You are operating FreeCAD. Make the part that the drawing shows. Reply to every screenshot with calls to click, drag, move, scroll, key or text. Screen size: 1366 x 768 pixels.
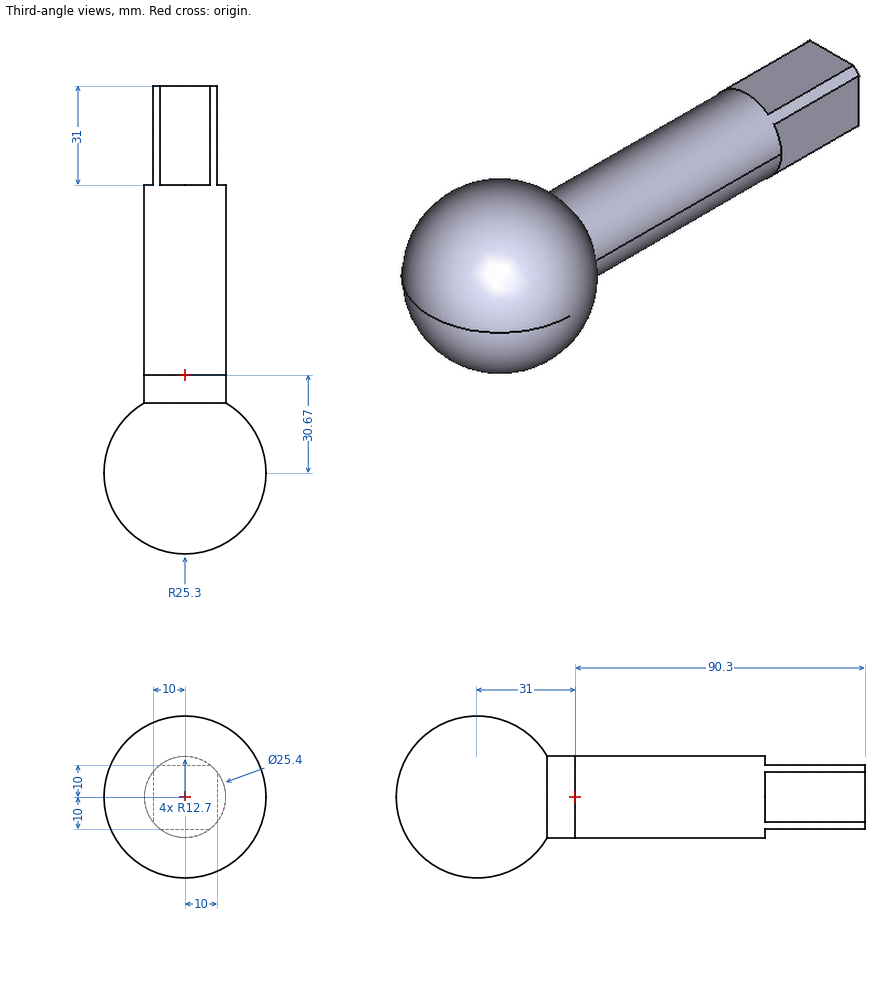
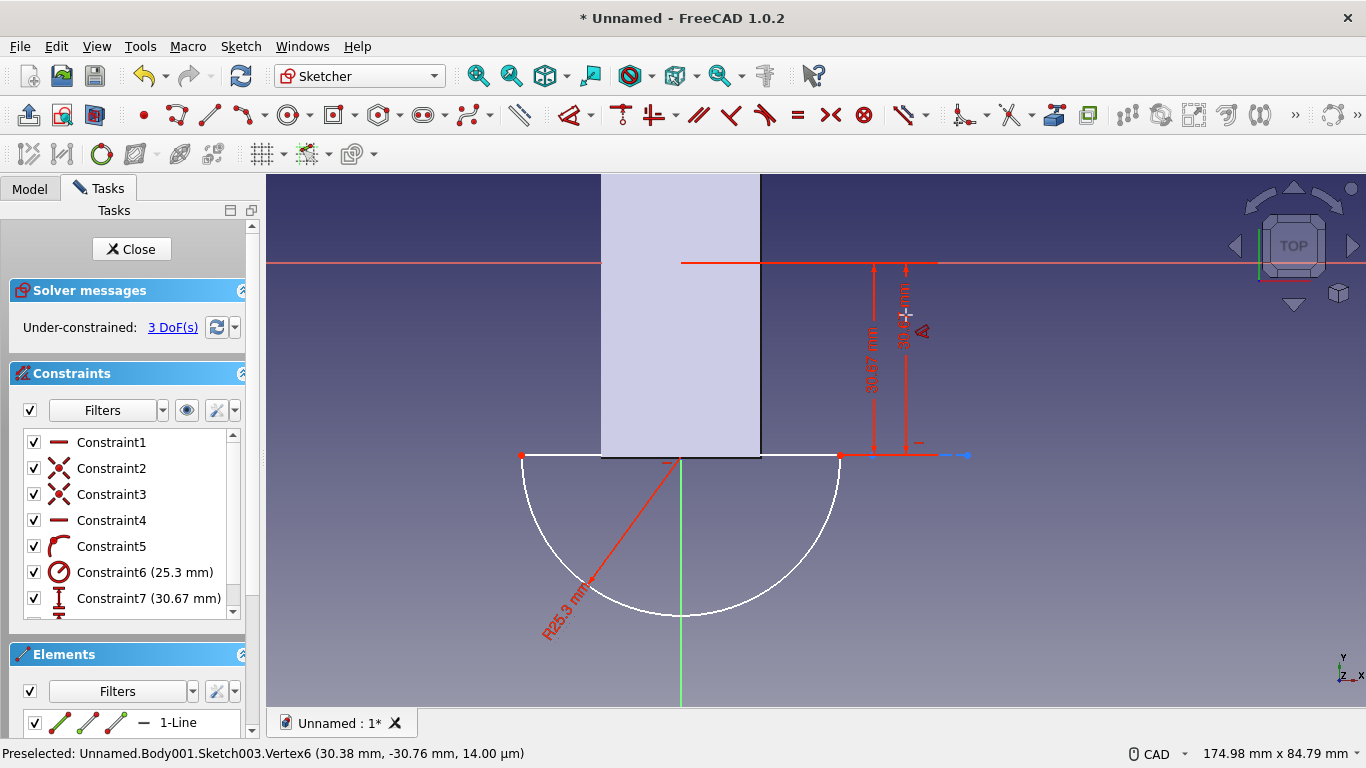
click(681, 457)
click(647, 360)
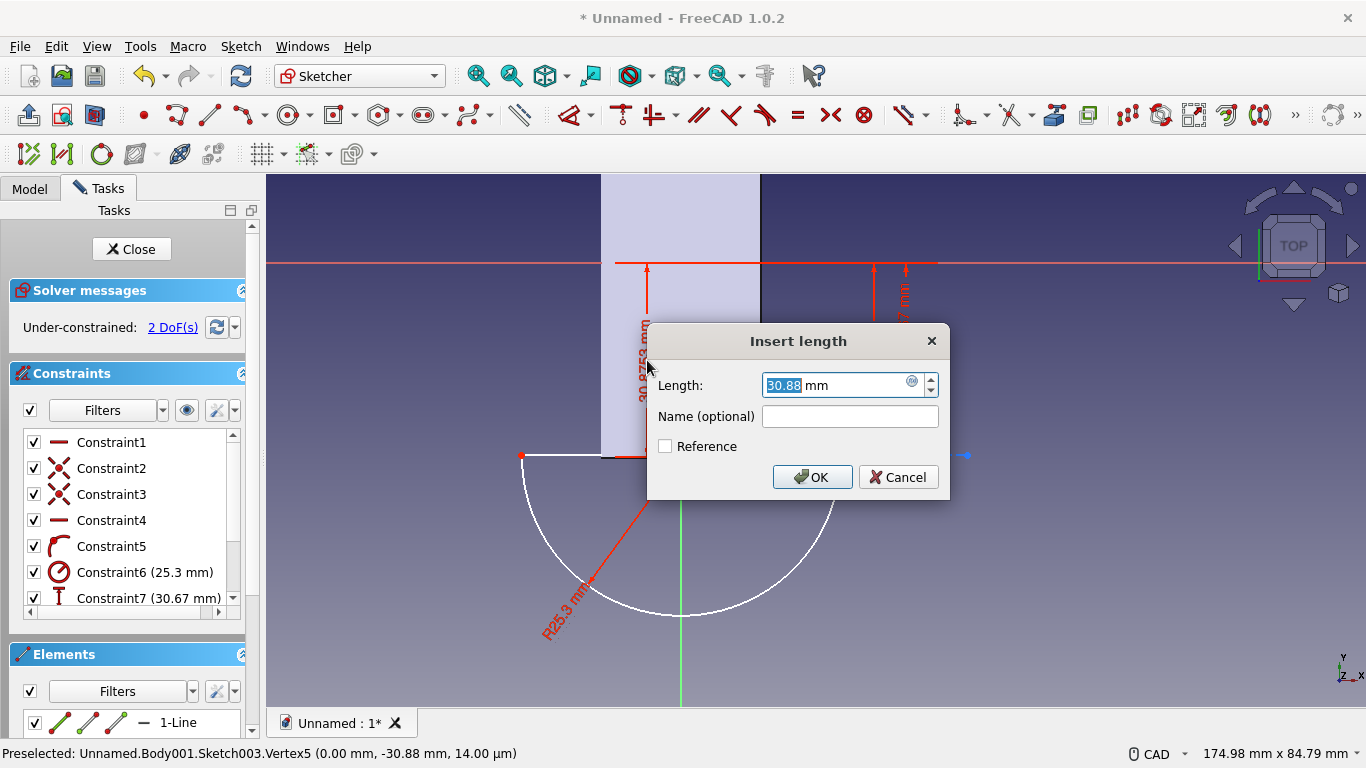
text(30.67)
key(Return)
key(Escape)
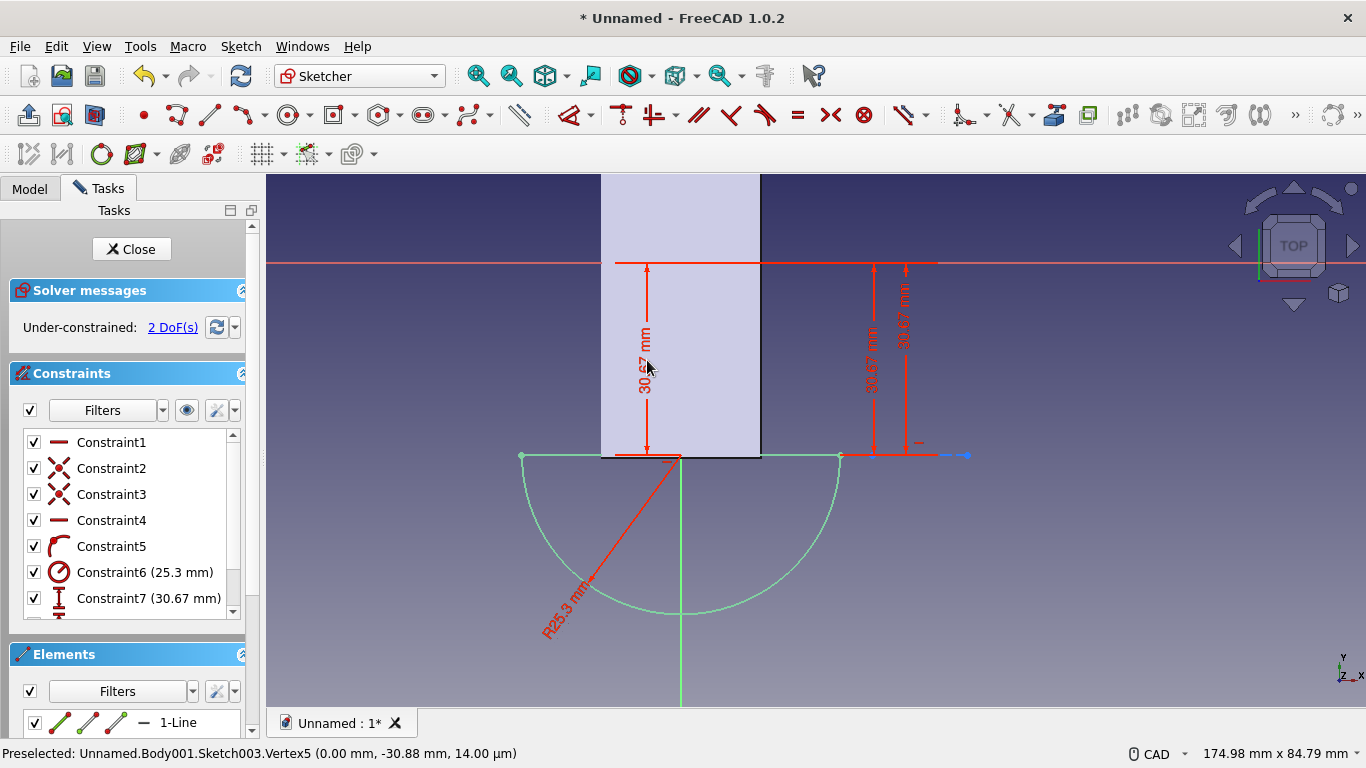
click(132, 249)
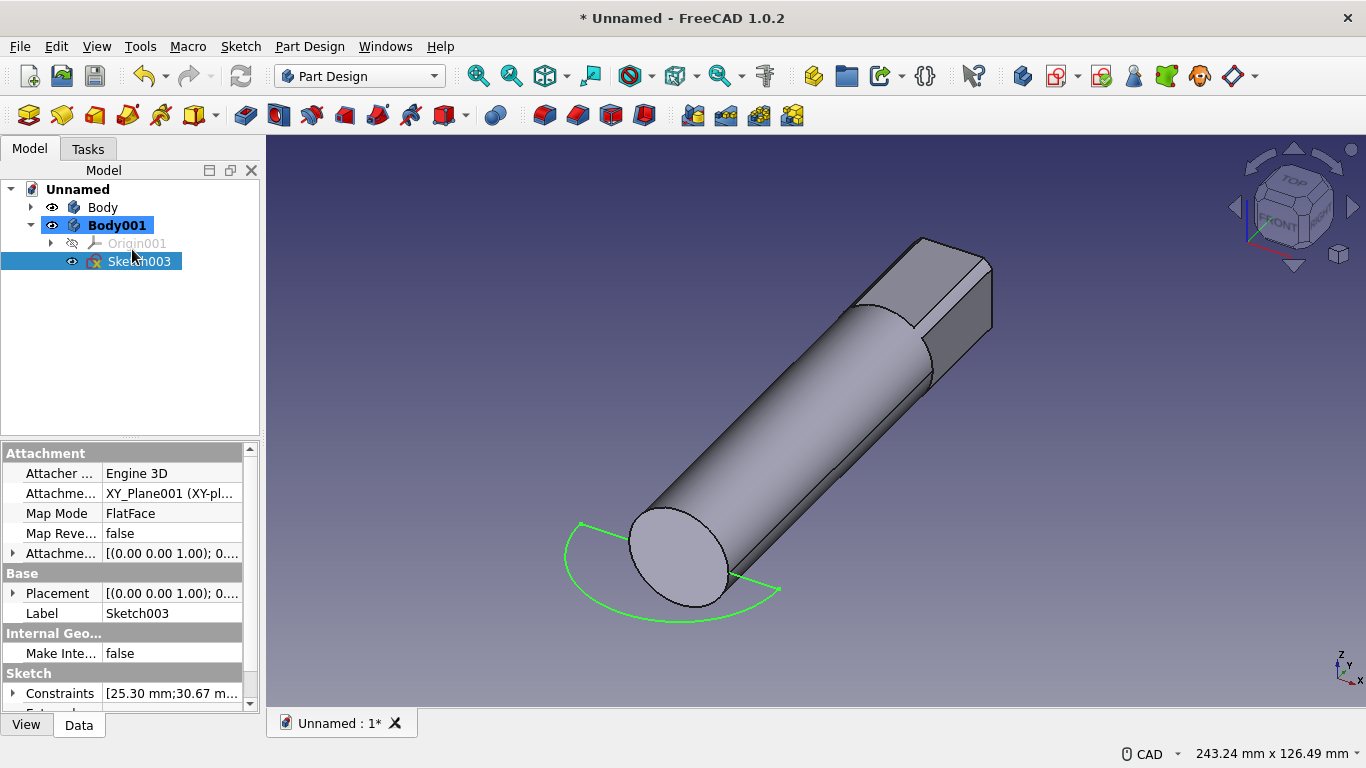
click(62, 116)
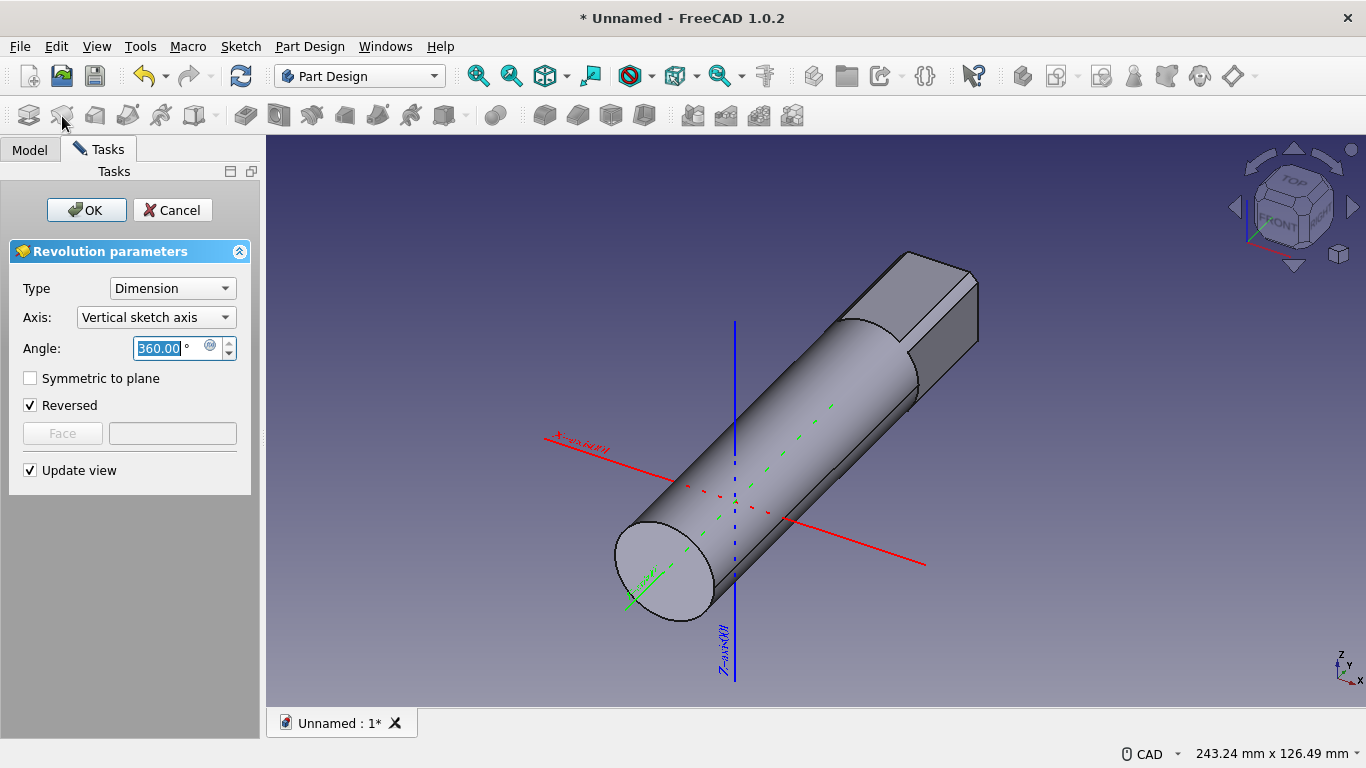
click(157, 318)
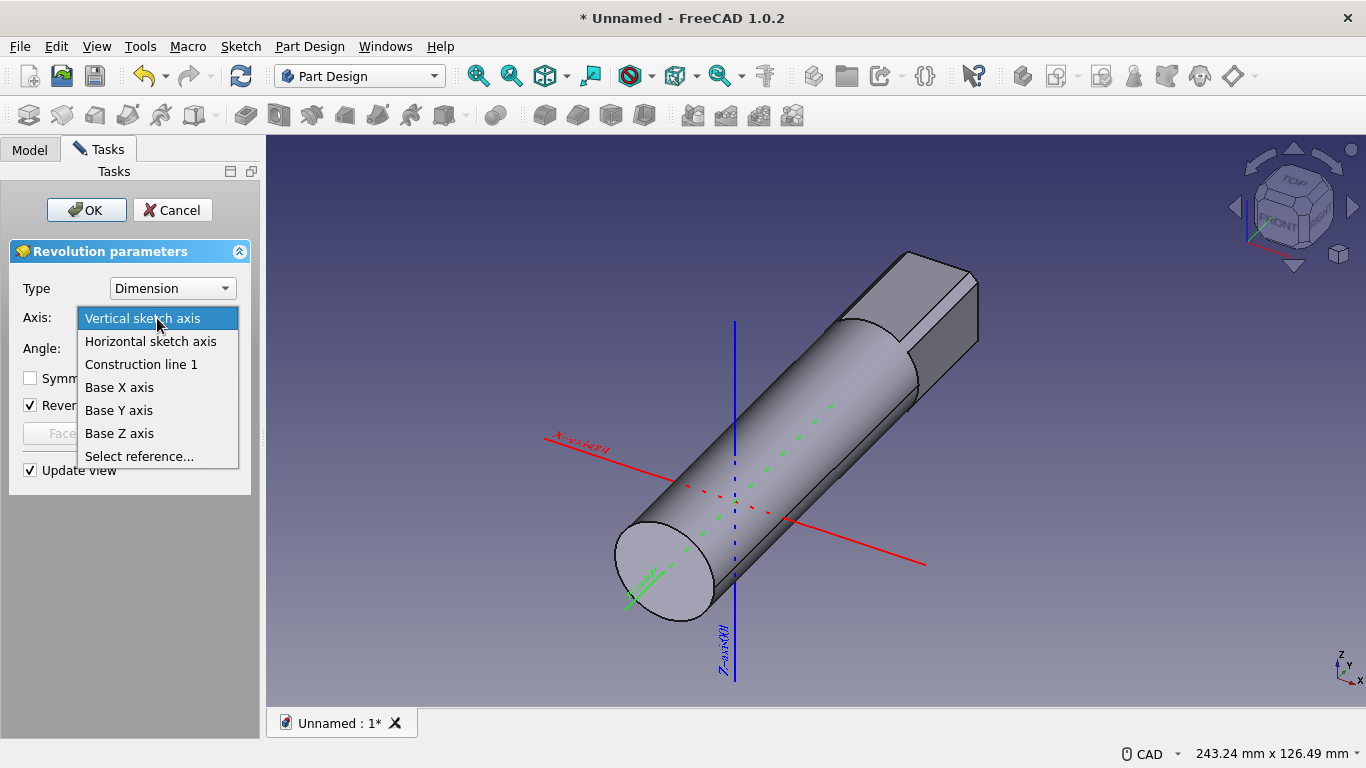
click(156, 364)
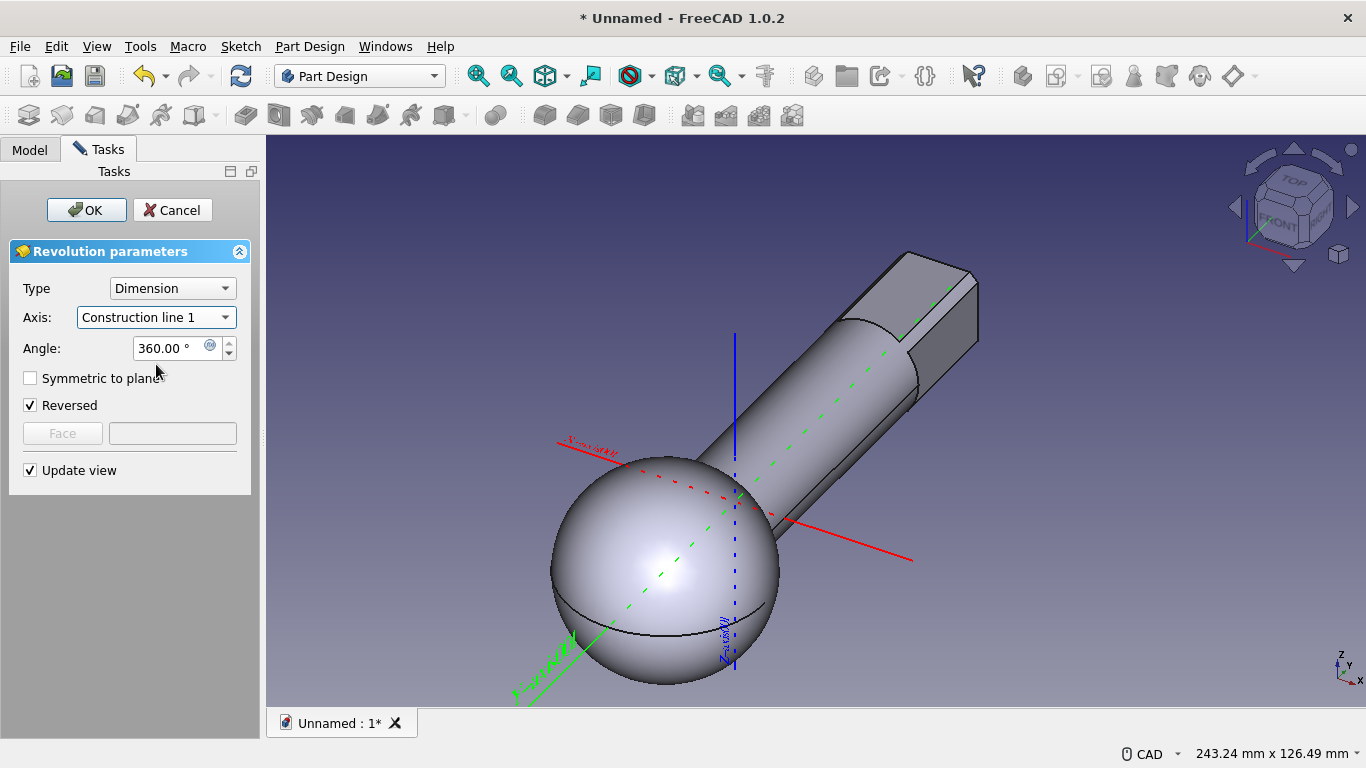
click(87, 210)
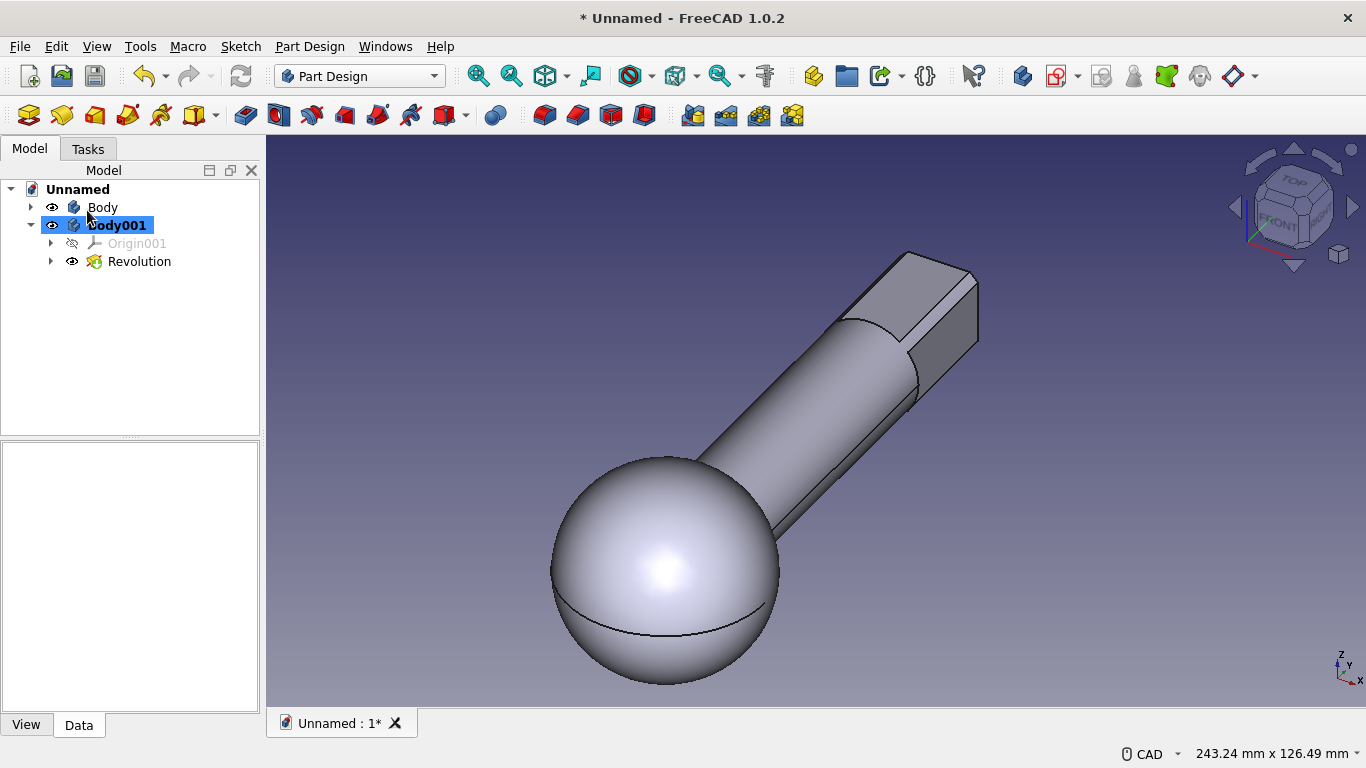
key(v)
key(f)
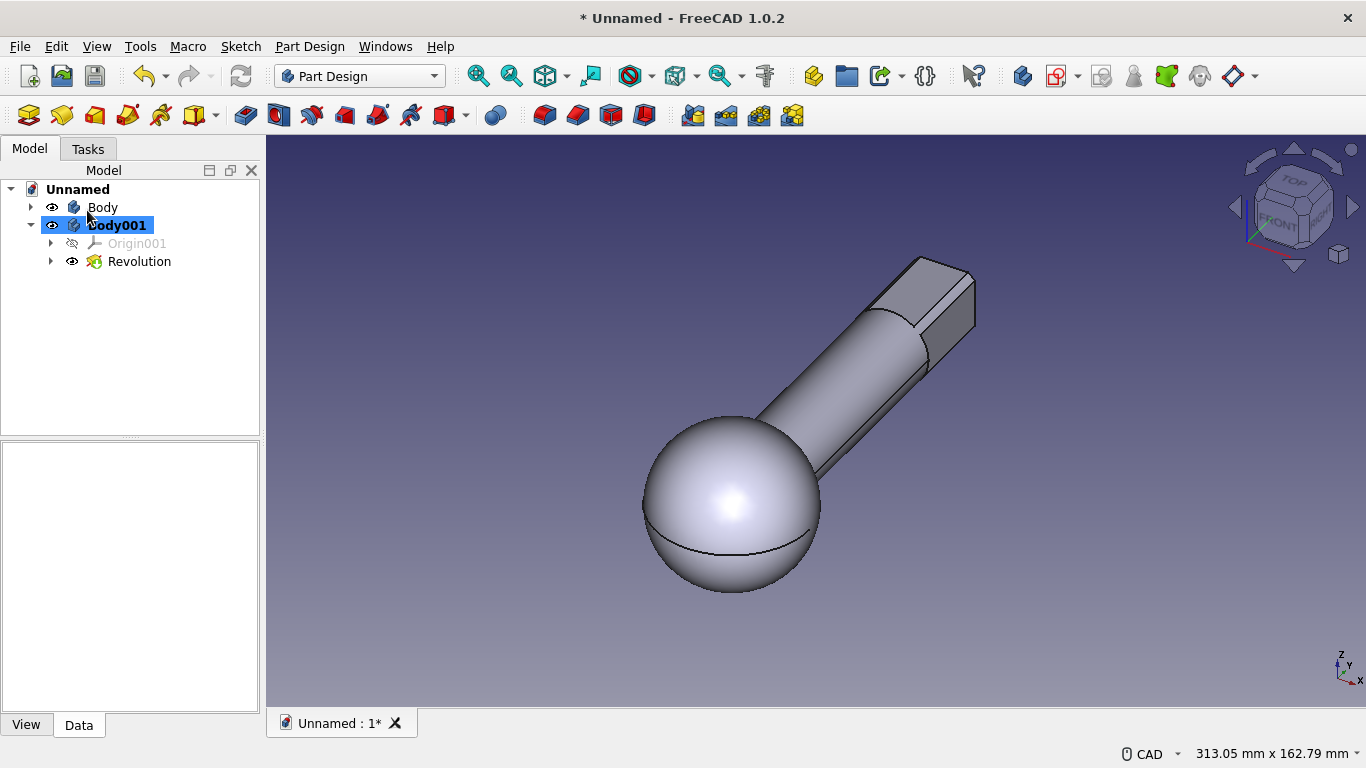
click(97, 207)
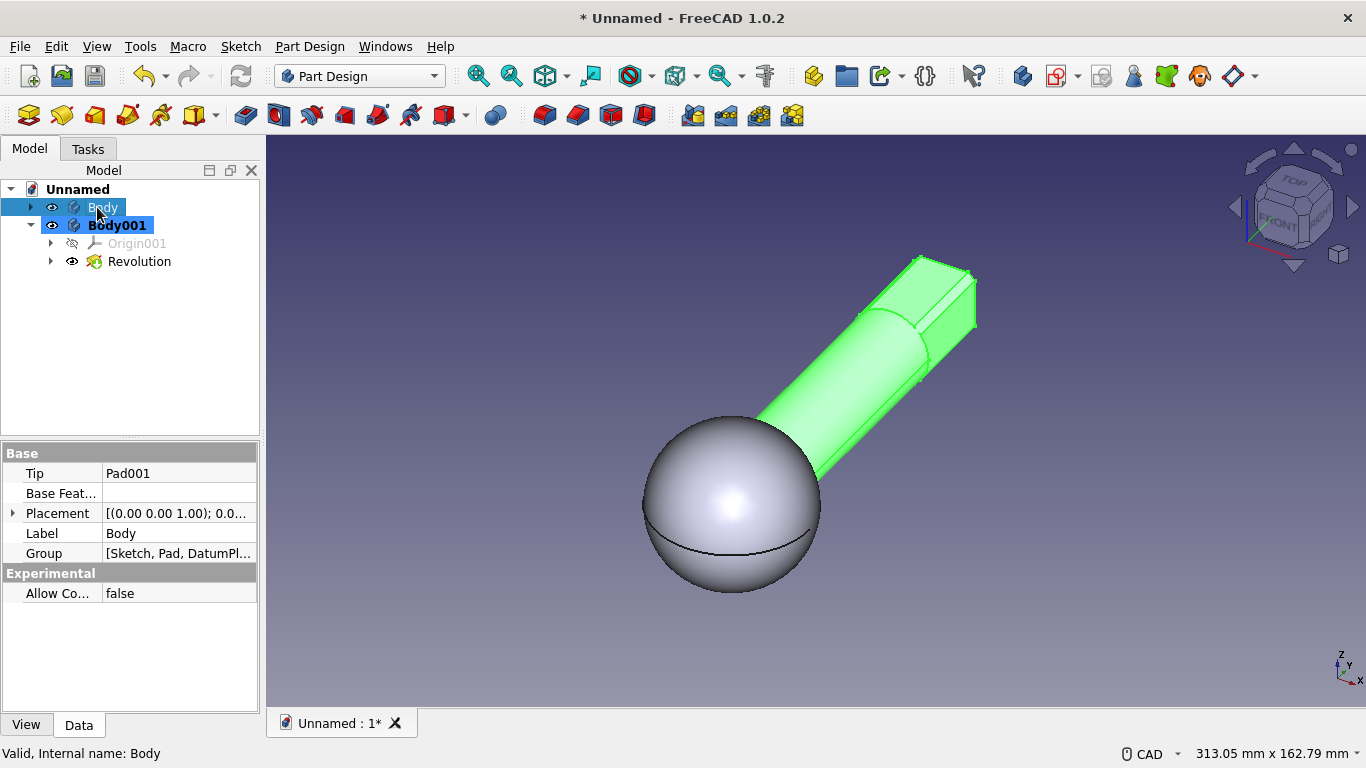
click(496, 116)